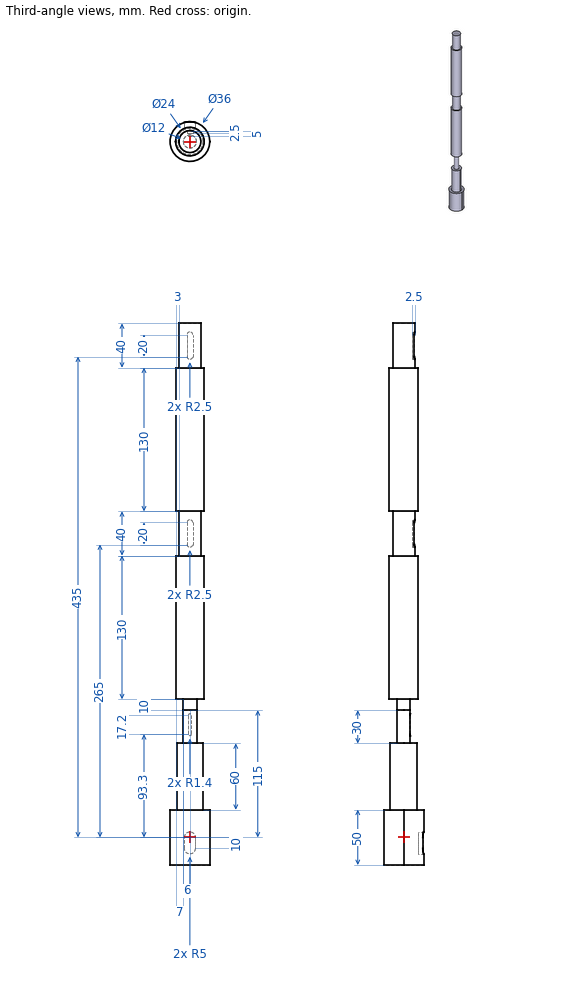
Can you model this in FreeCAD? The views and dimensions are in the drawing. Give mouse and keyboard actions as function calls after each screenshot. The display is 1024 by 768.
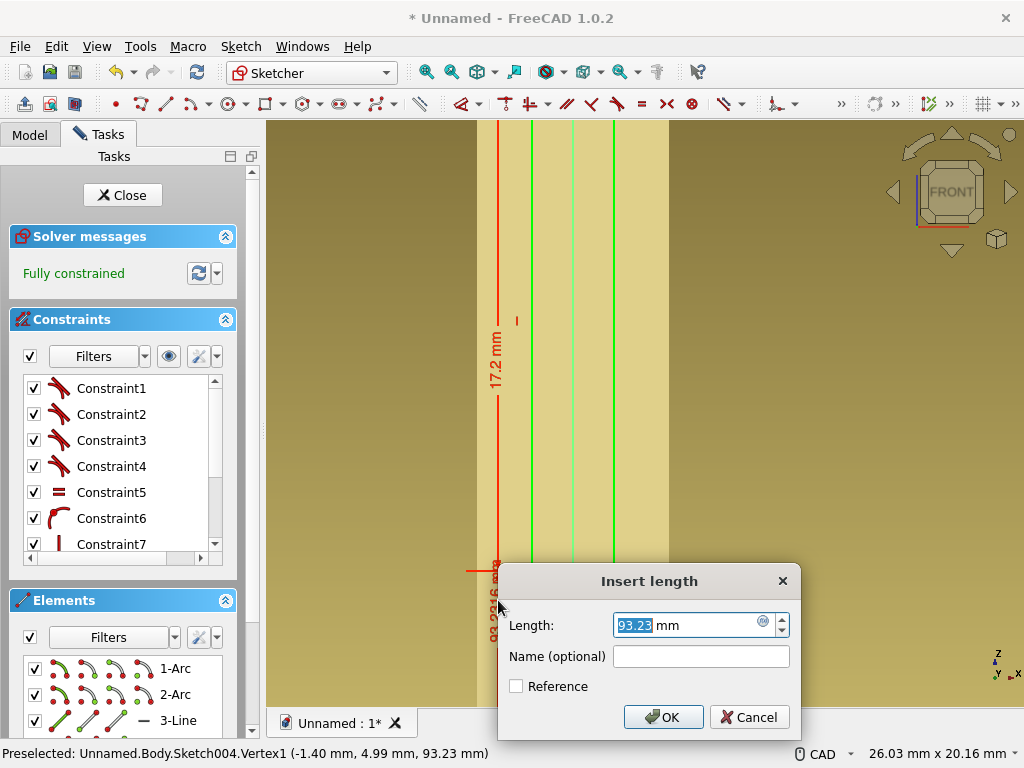
text(93.3)
key(Return)
key(Escape)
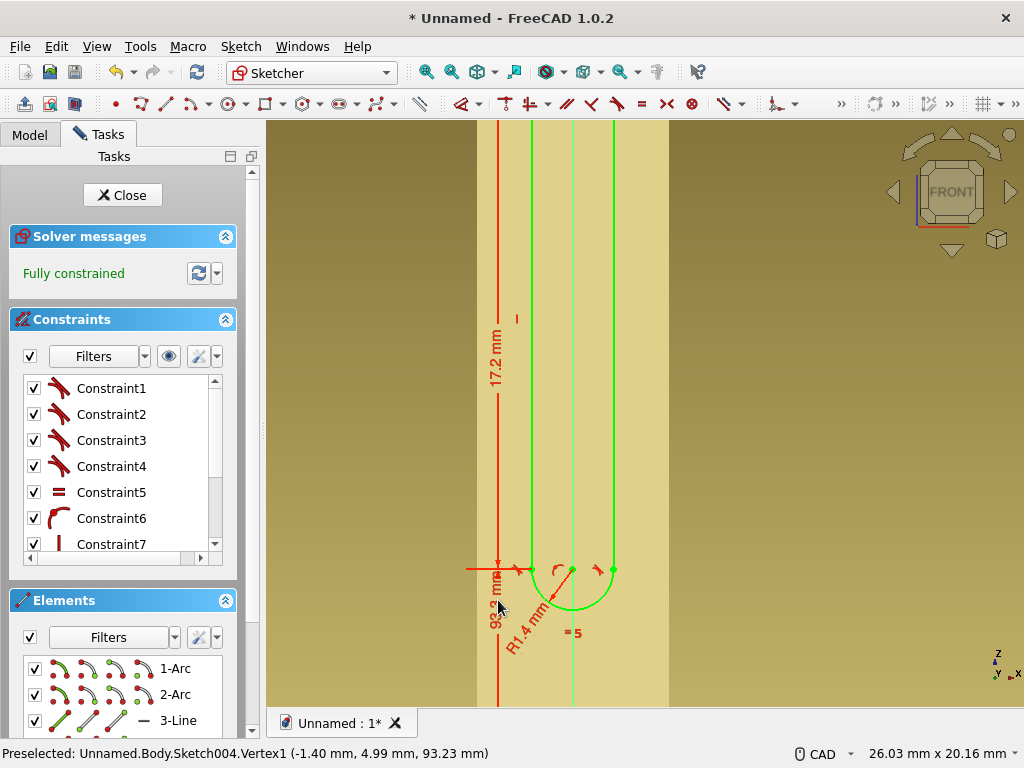
click(123, 195)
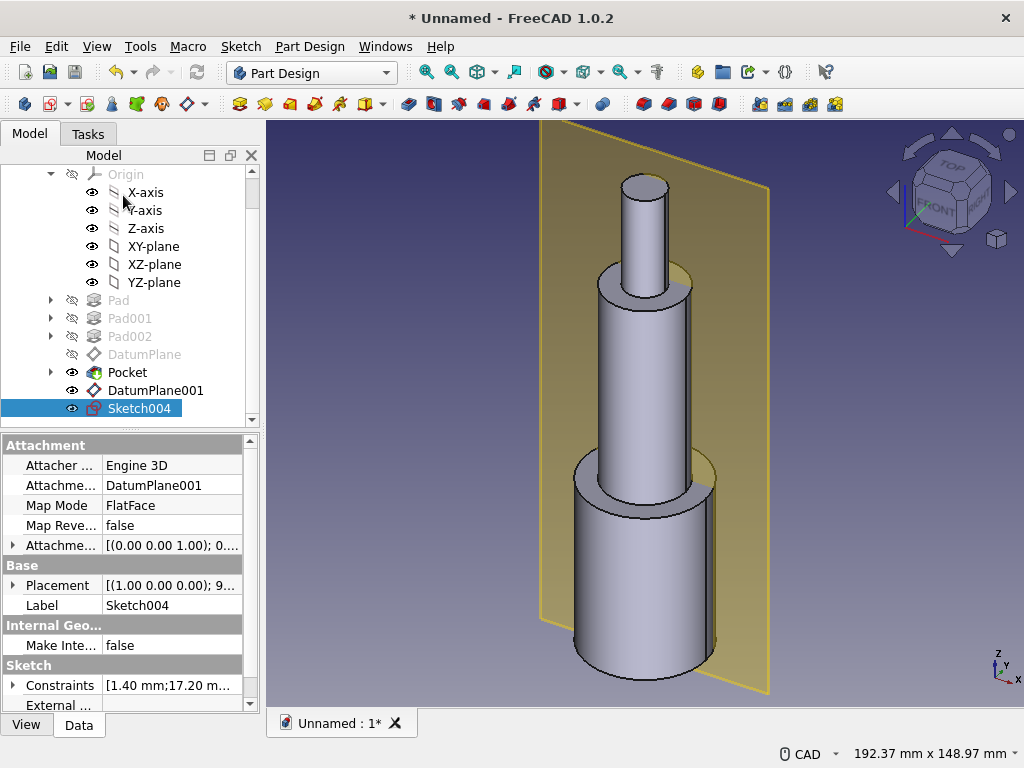
click(409, 104)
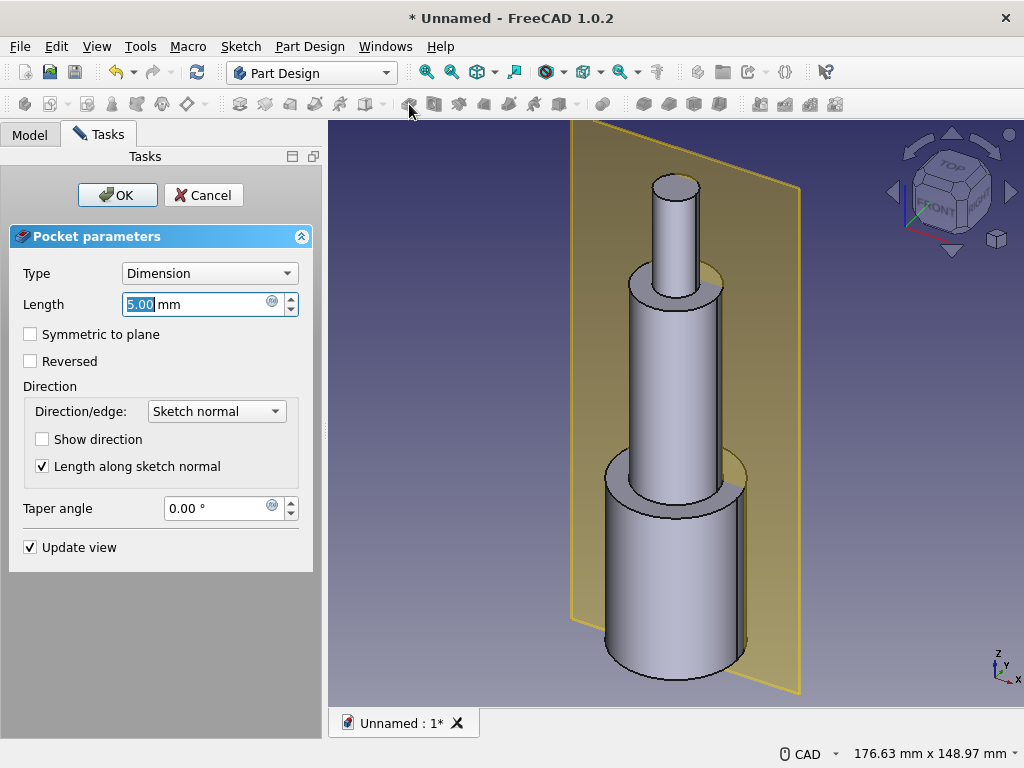
text(5)
key(Tab)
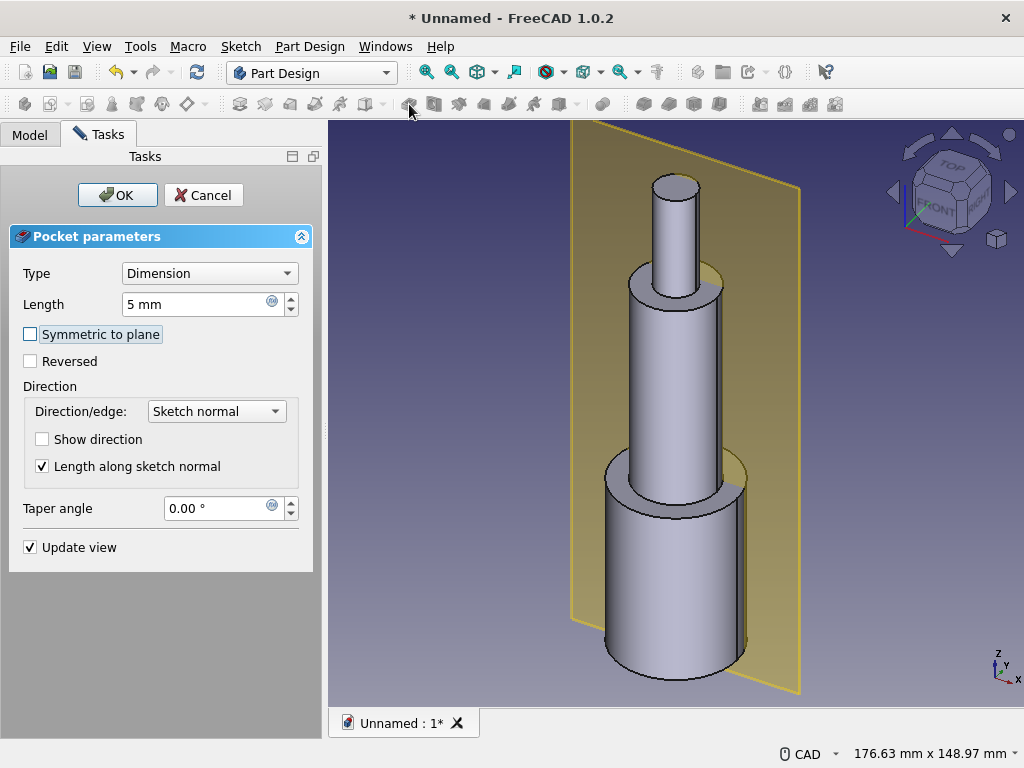
click(118, 195)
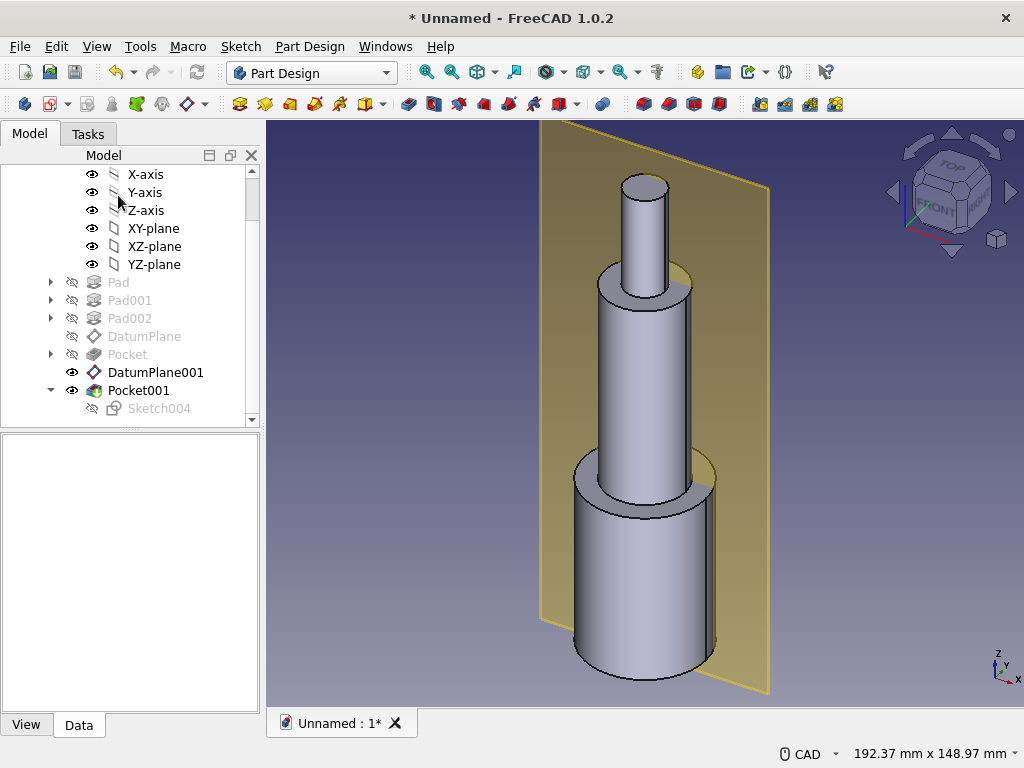
click(117, 372)
key(space)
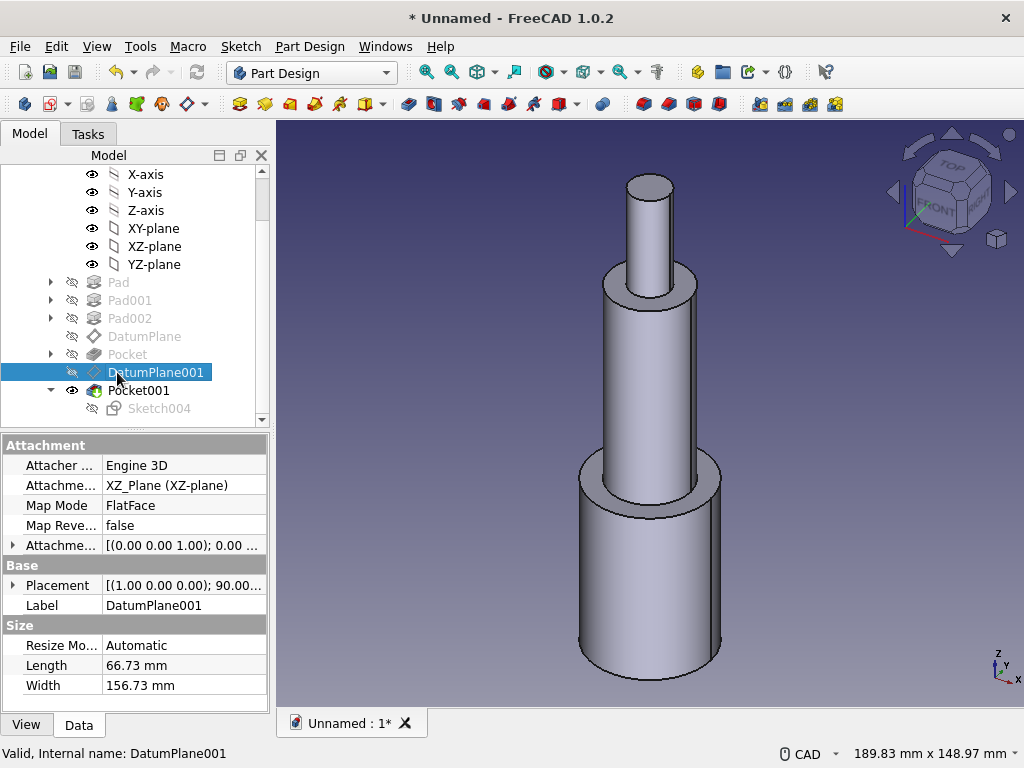
click(316, 667)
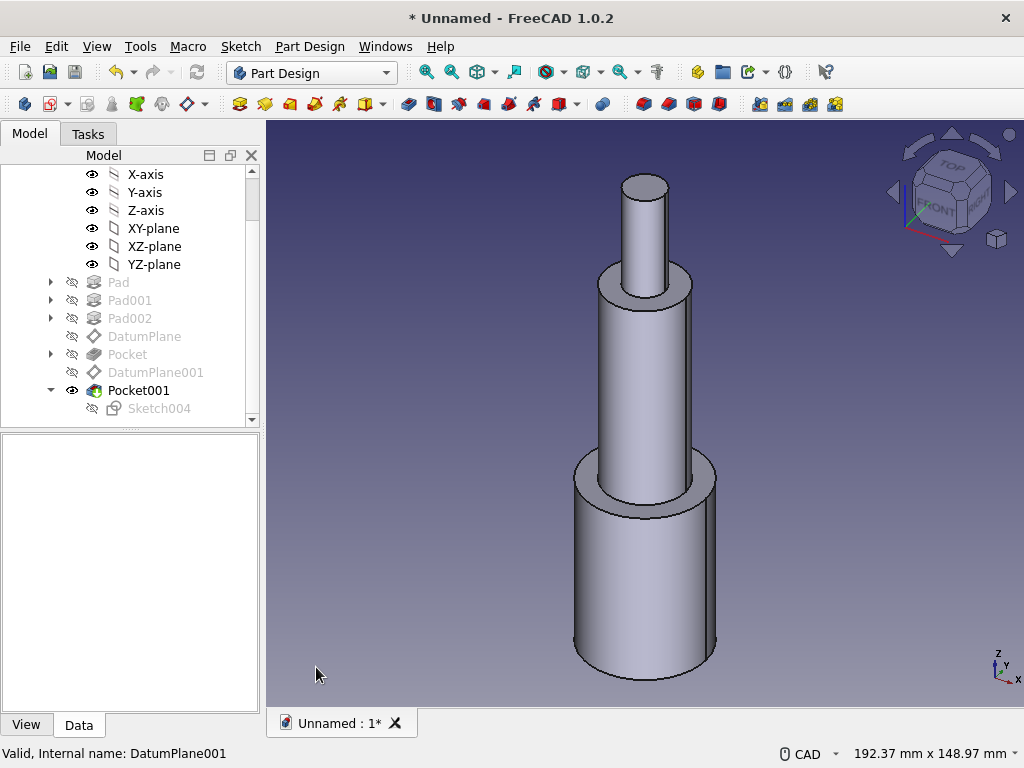
click(50, 104)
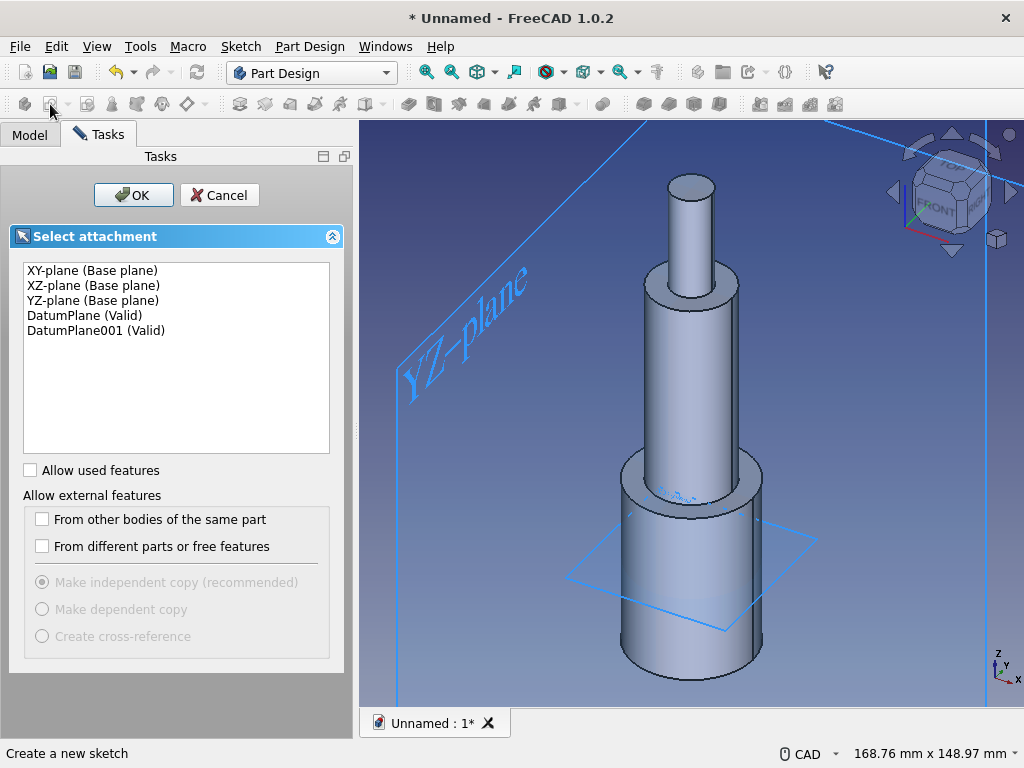
click(84, 286)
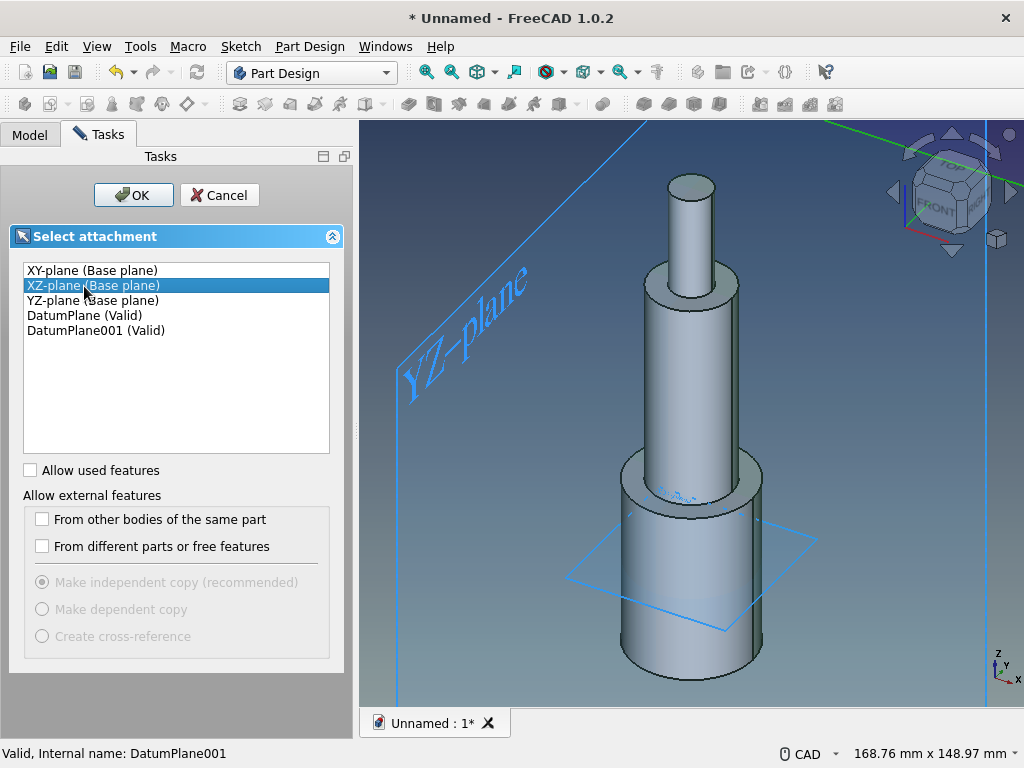
click(134, 195)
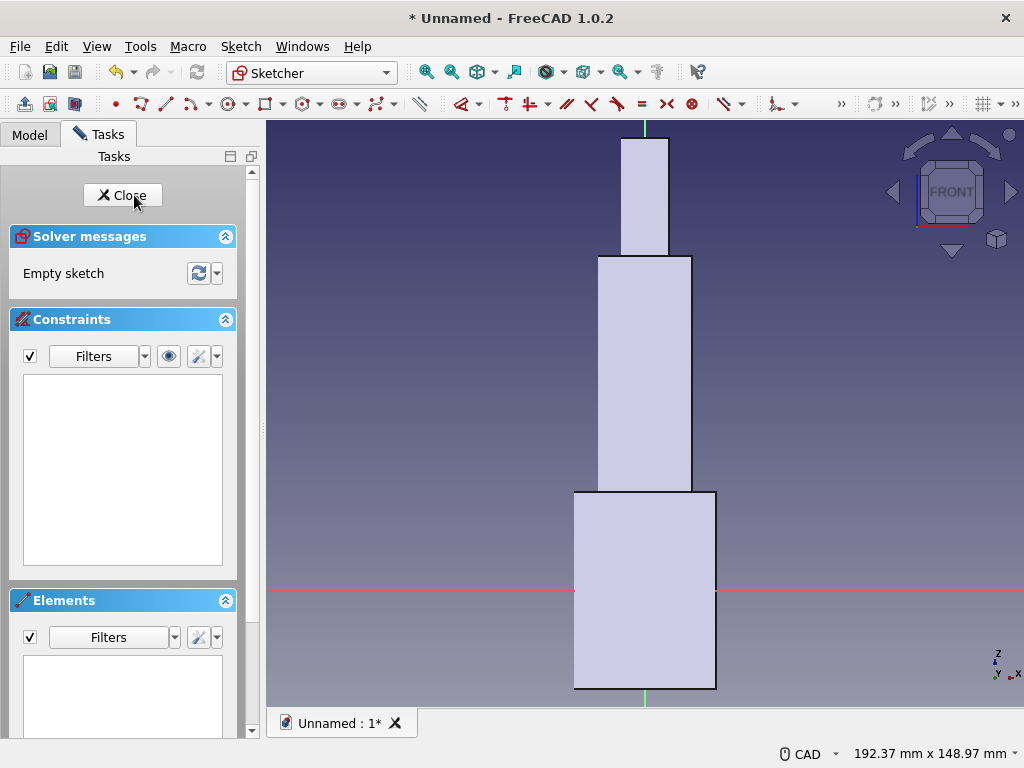
click(75, 104)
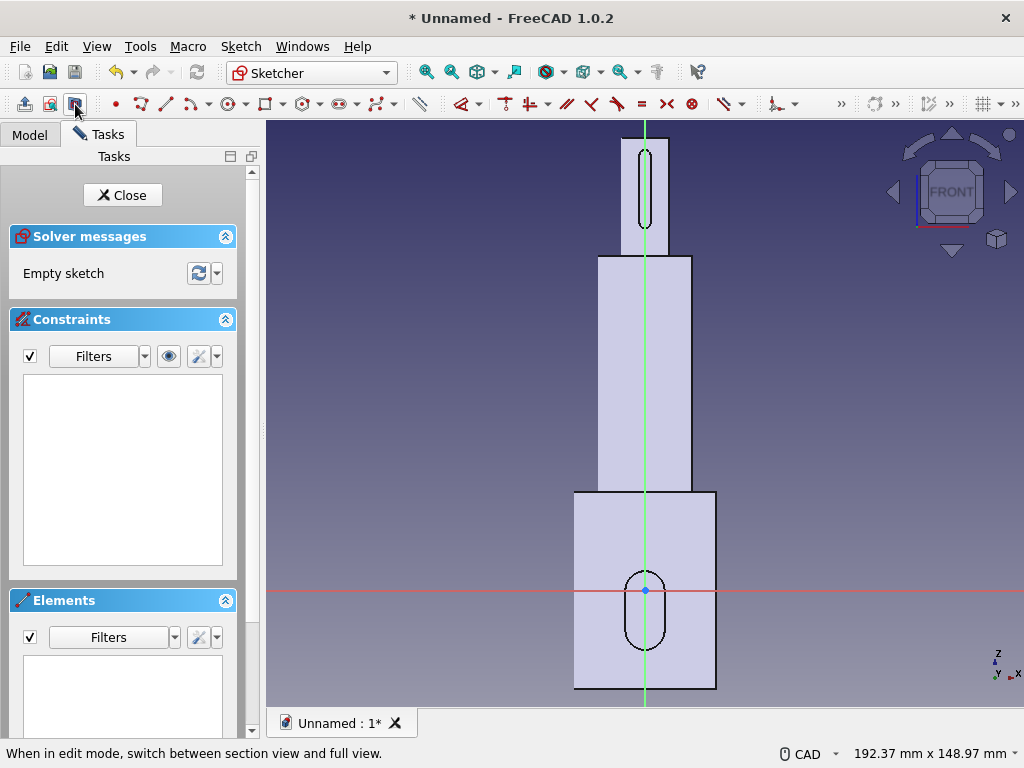
scroll(566, 600, down, 8)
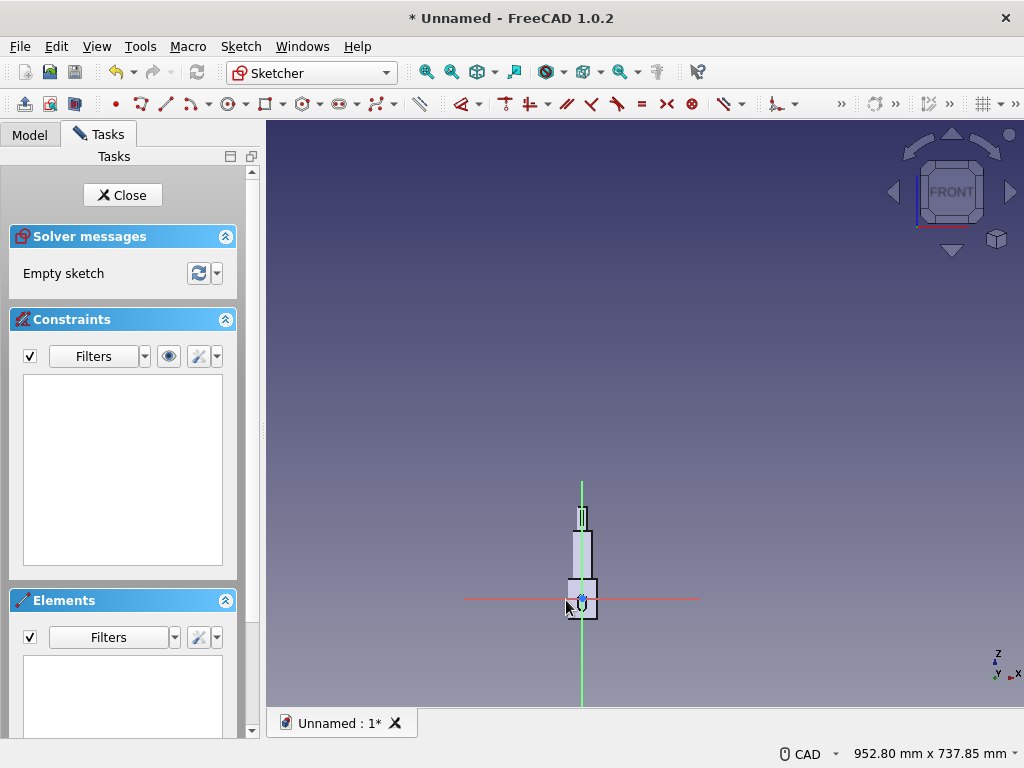
click(141, 104)